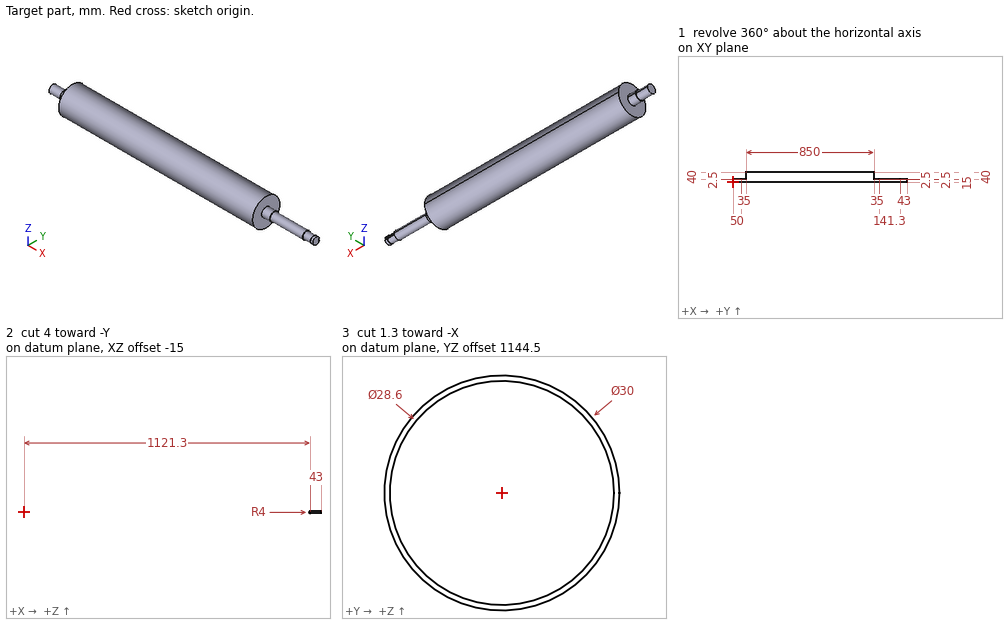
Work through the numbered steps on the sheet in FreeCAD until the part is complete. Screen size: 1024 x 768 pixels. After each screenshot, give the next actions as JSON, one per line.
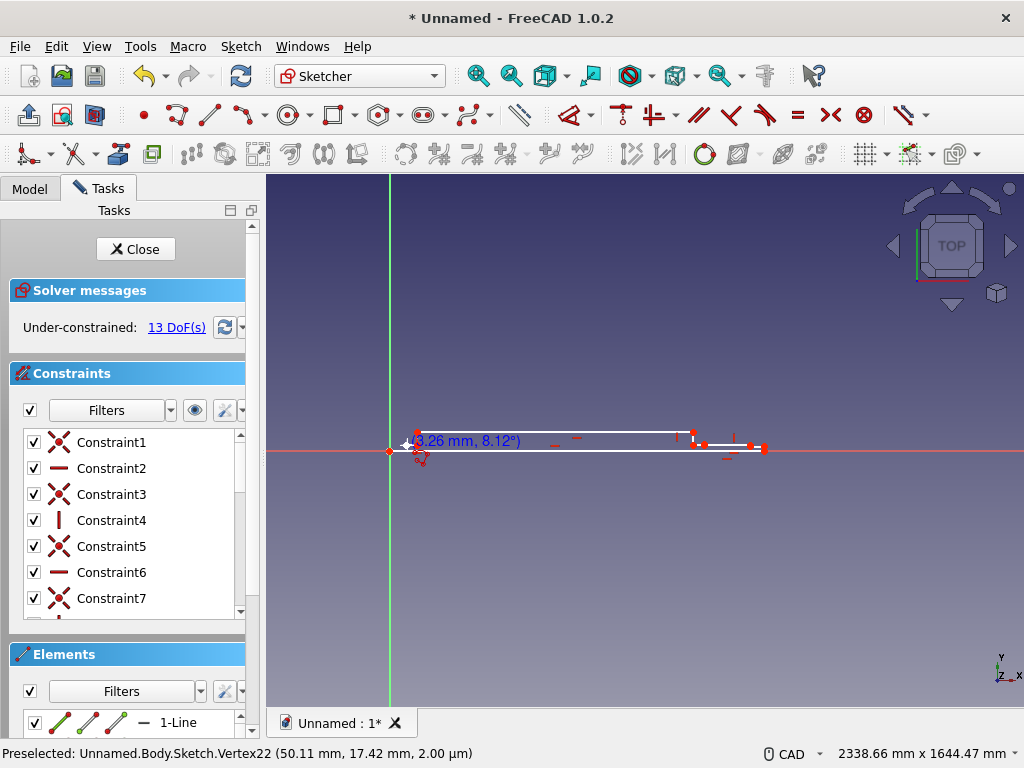
{"action": "scroll", "coordinate": [390, 445], "scroll_direction": "up", "scroll_amount": 6}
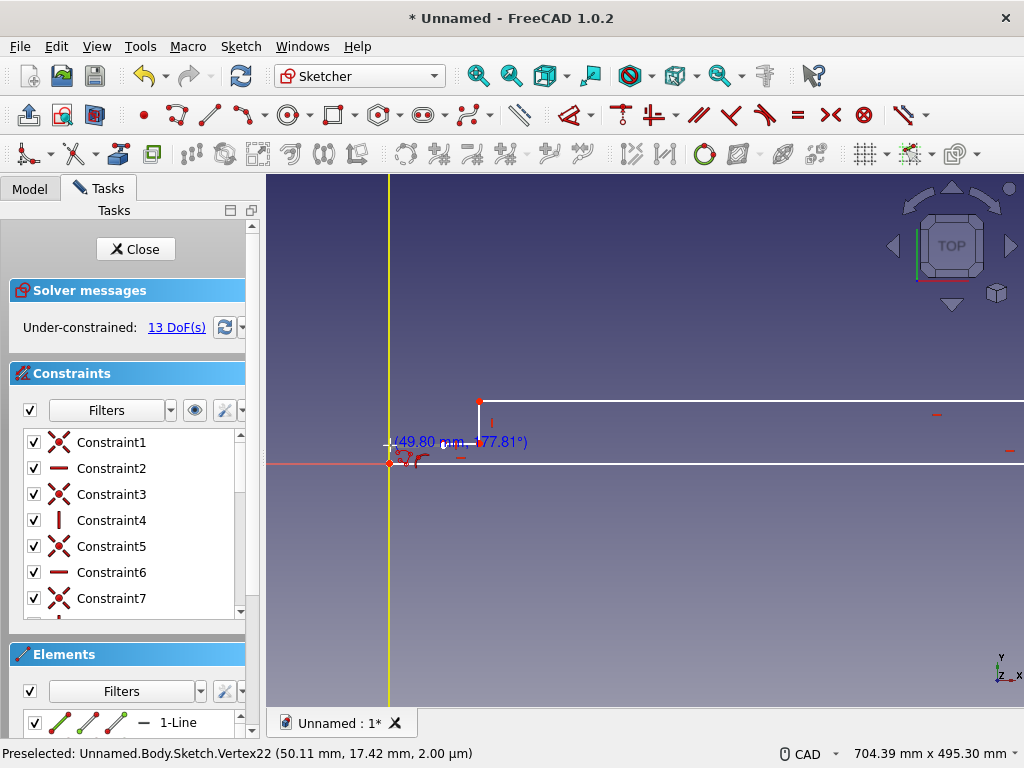
{"action": "left_click", "coordinate": [398, 445]}
{"action": "left_click", "coordinate": [389, 464]}
{"action": "key", "text": "Escape"}
{"action": "key", "text": "Escape"}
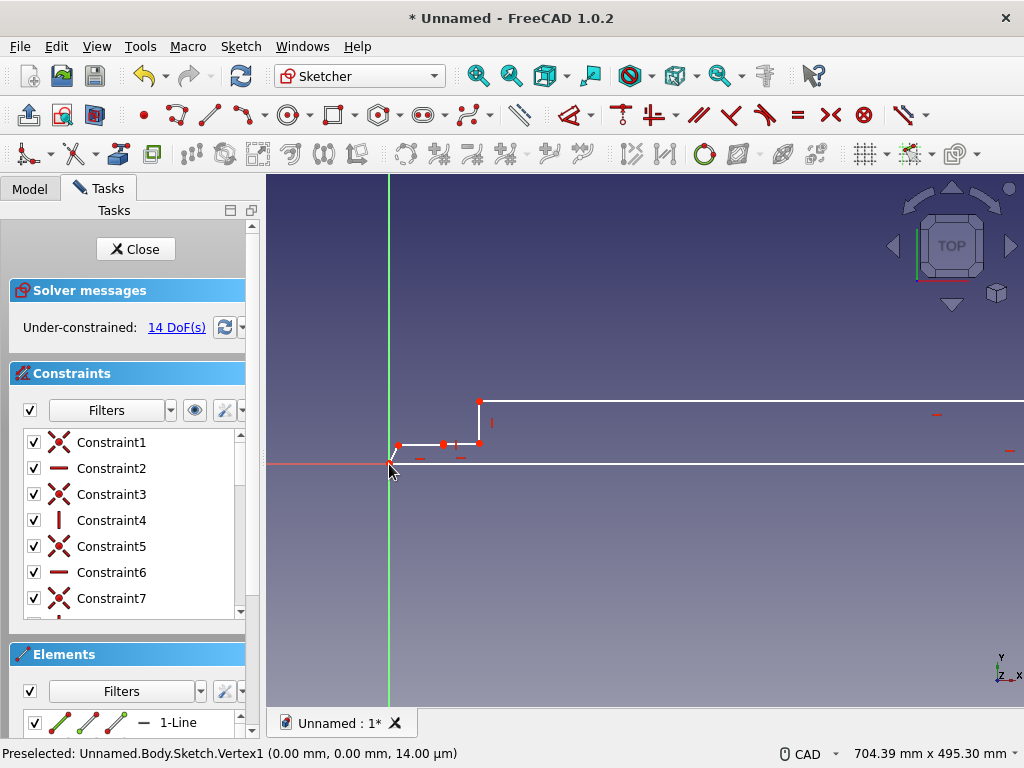
{"action": "scroll", "coordinate": [389, 444], "scroll_direction": "down", "scroll_amount": 6}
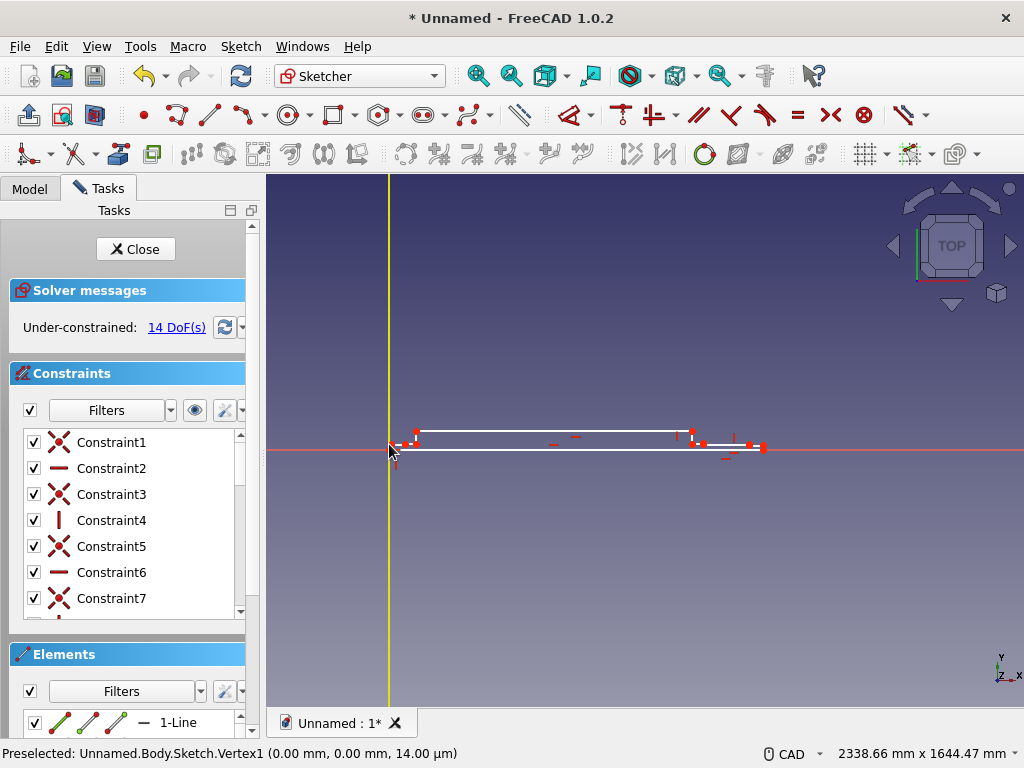
{"action": "scroll", "coordinate": [700, 444], "scroll_direction": "up", "scroll_amount": 7}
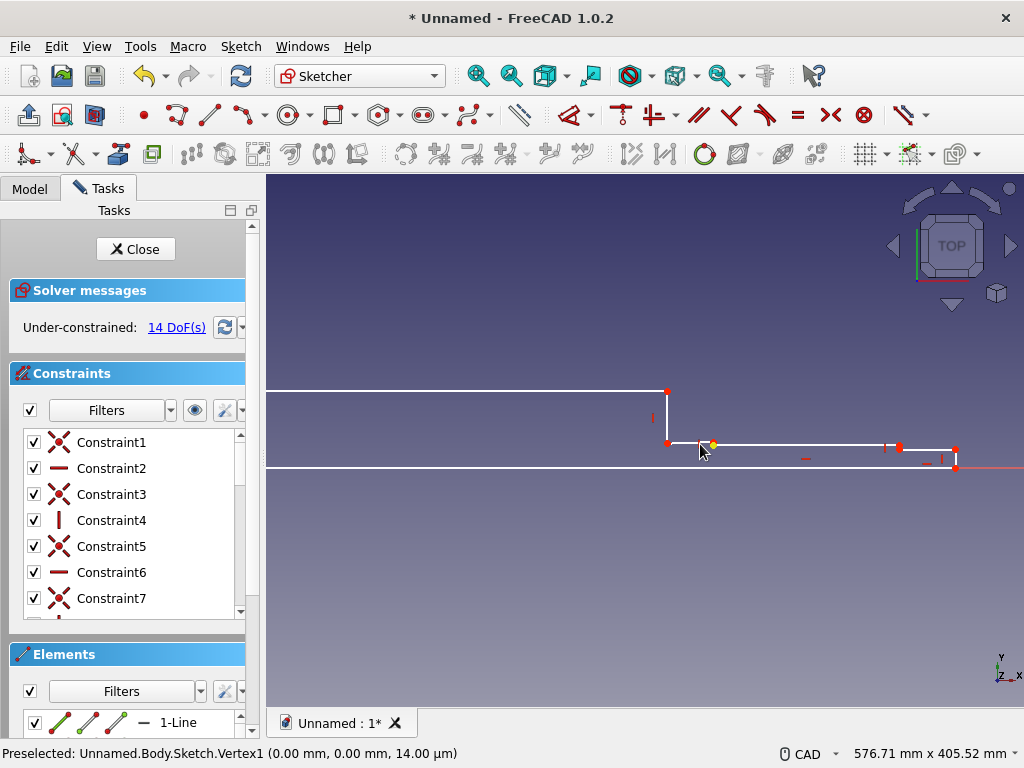
{"action": "left_click", "coordinate": [681, 443]}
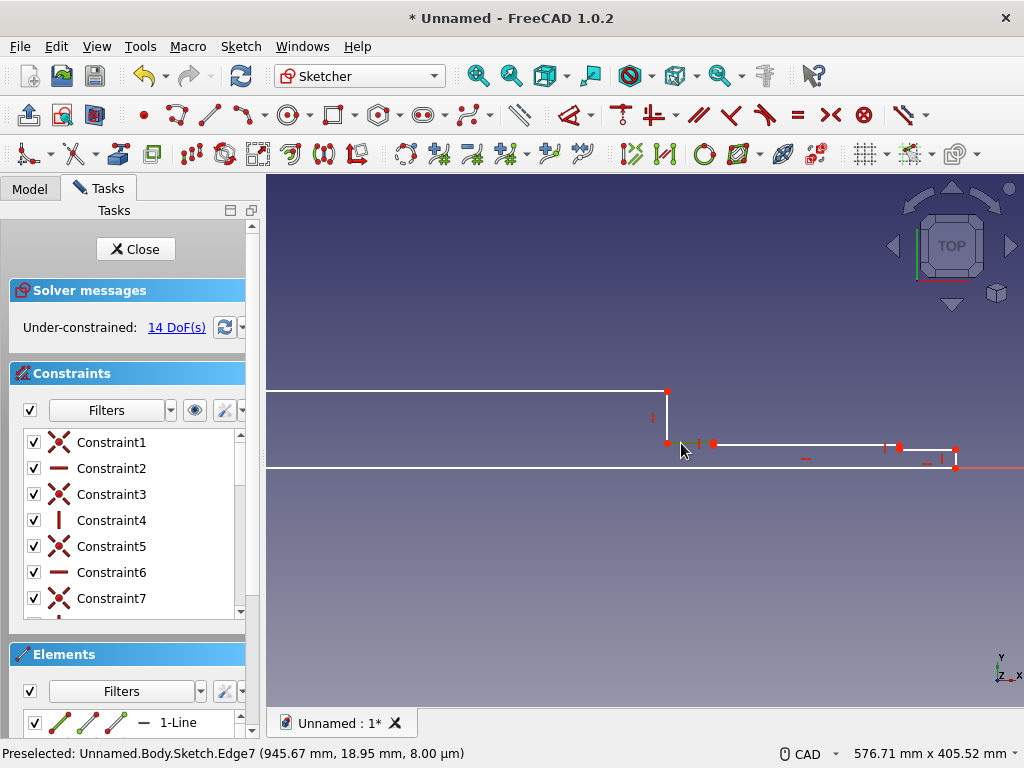
{"action": "key", "text": "h"}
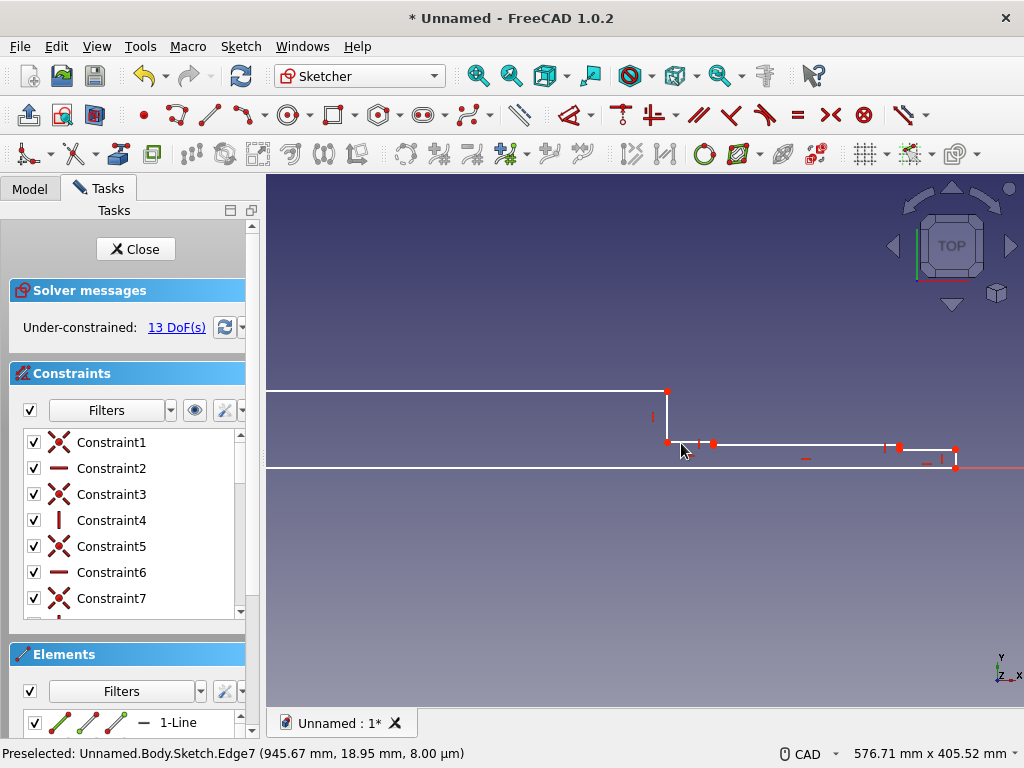
{"action": "scroll", "coordinate": [701, 444], "scroll_direction": "down", "scroll_amount": 7}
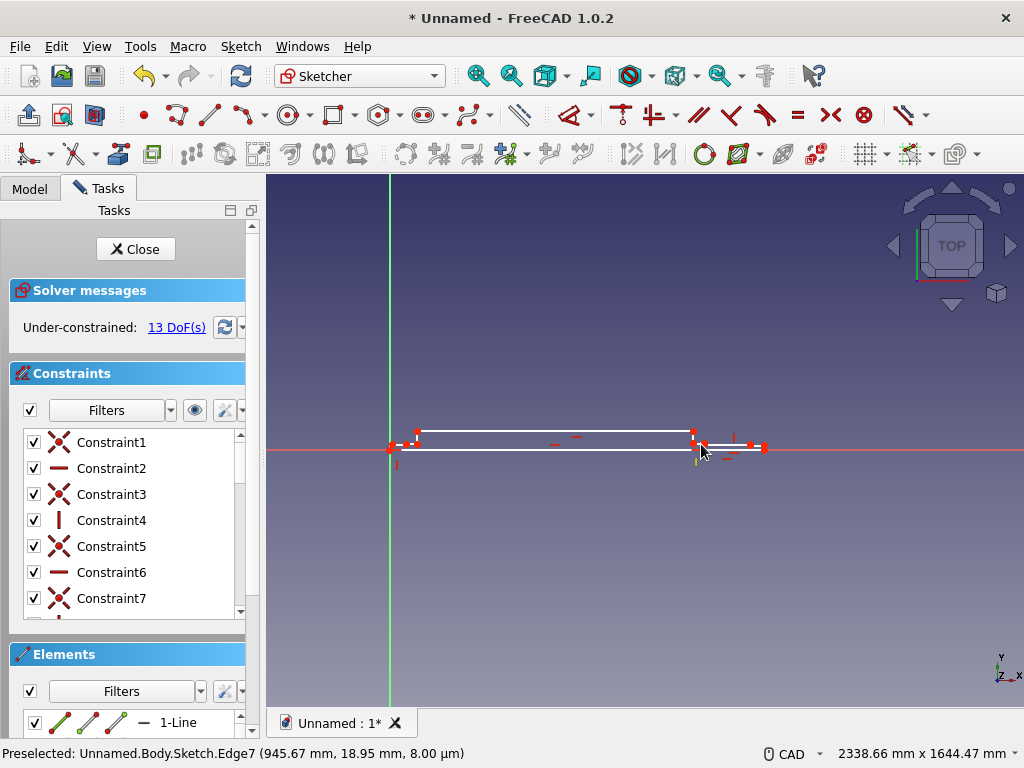
{"action": "scroll", "coordinate": [392, 446], "scroll_direction": "up", "scroll_amount": 11}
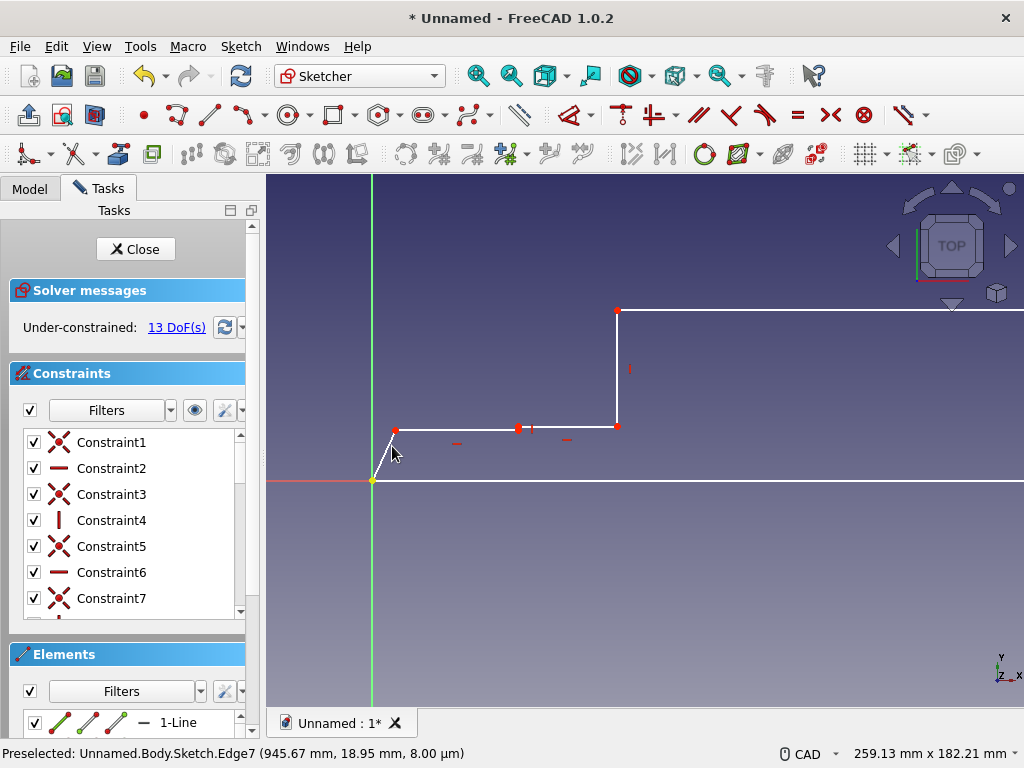
{"action": "left_click", "coordinate": [389, 445]}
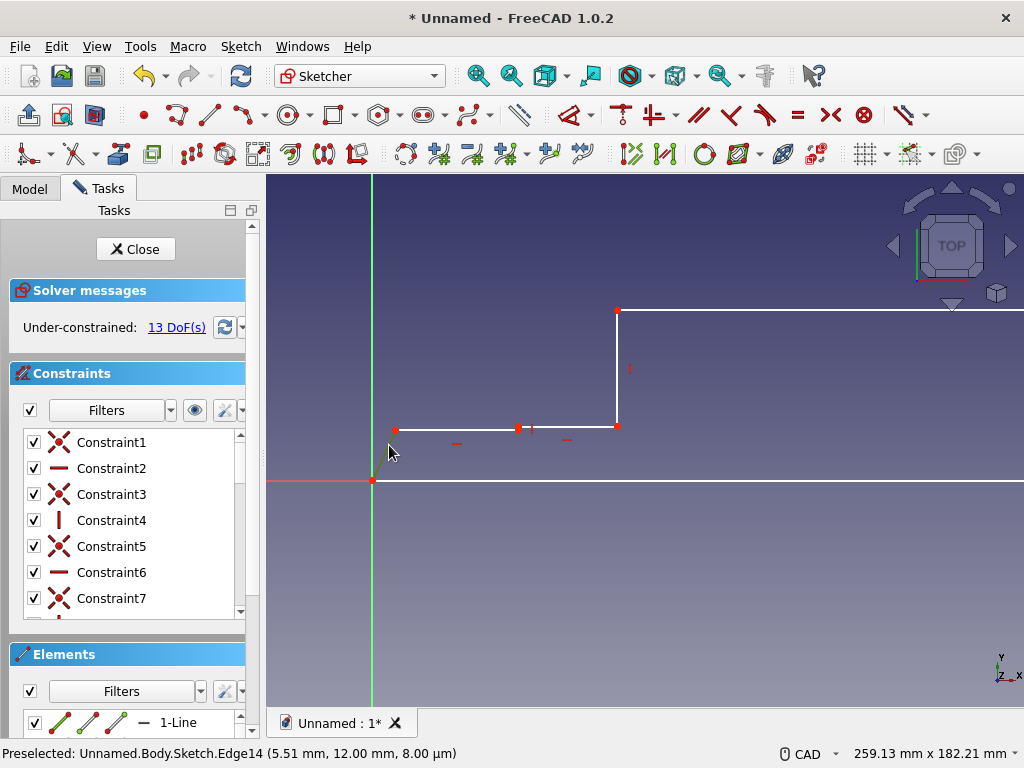
{"action": "left_click", "coordinate": [676, 116]}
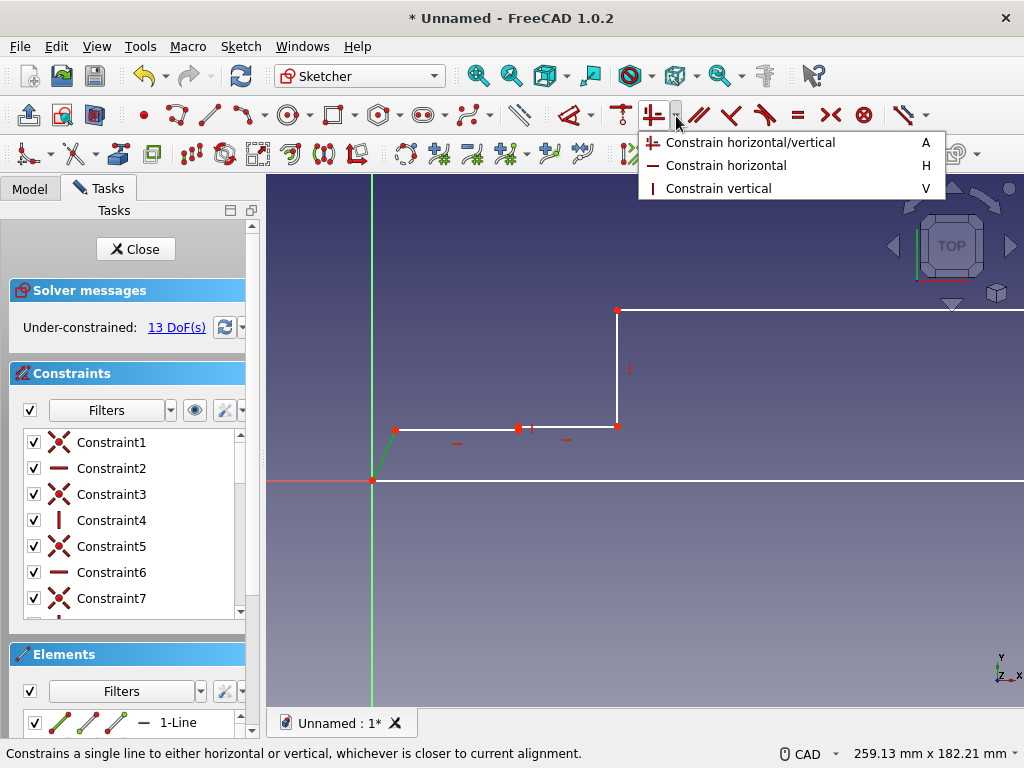
{"action": "left_click", "coordinate": [792, 188]}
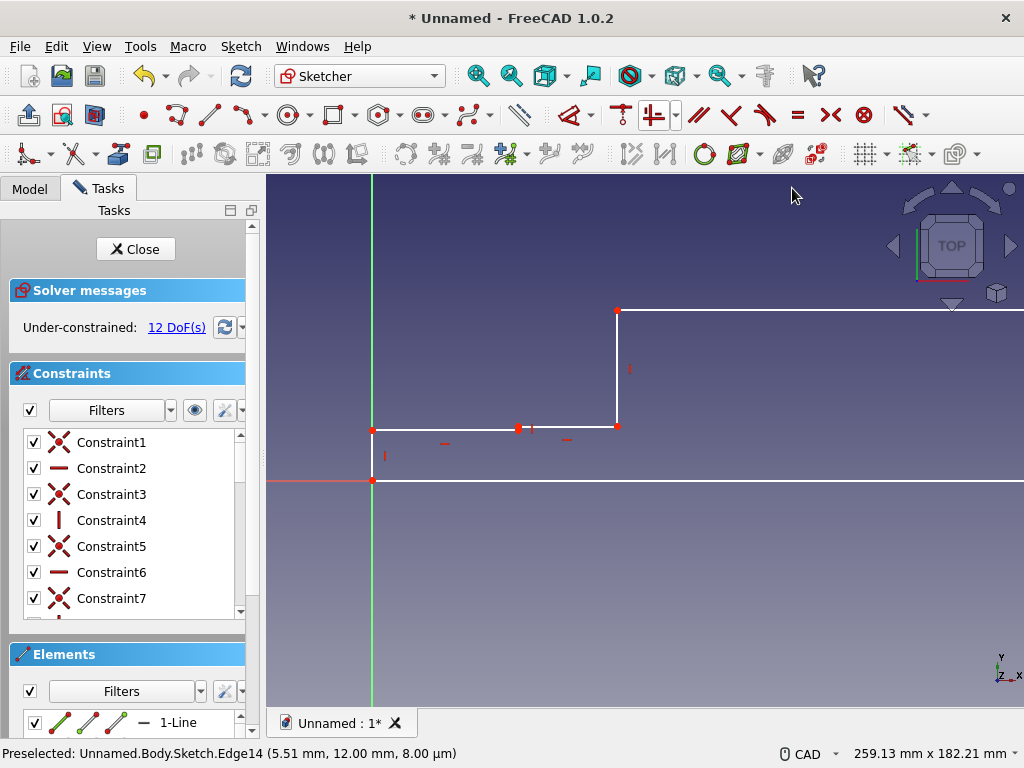
{"action": "key", "text": "d"}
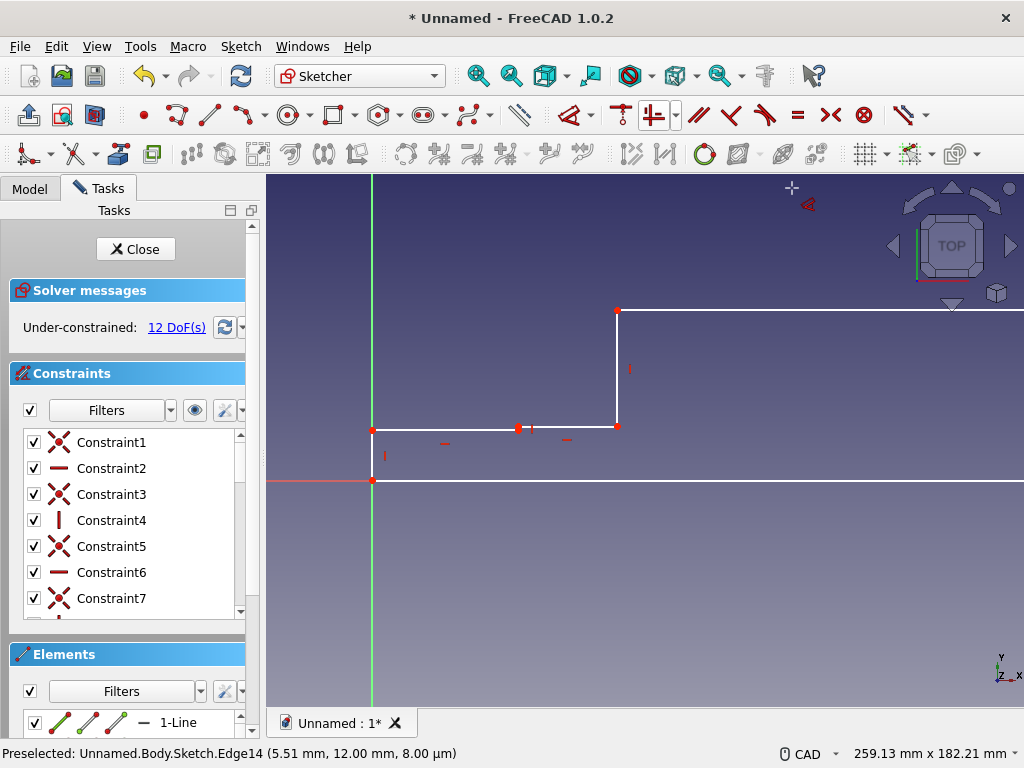
{"action": "scroll", "coordinate": [392, 446], "scroll_direction": "down", "scroll_amount": 11}